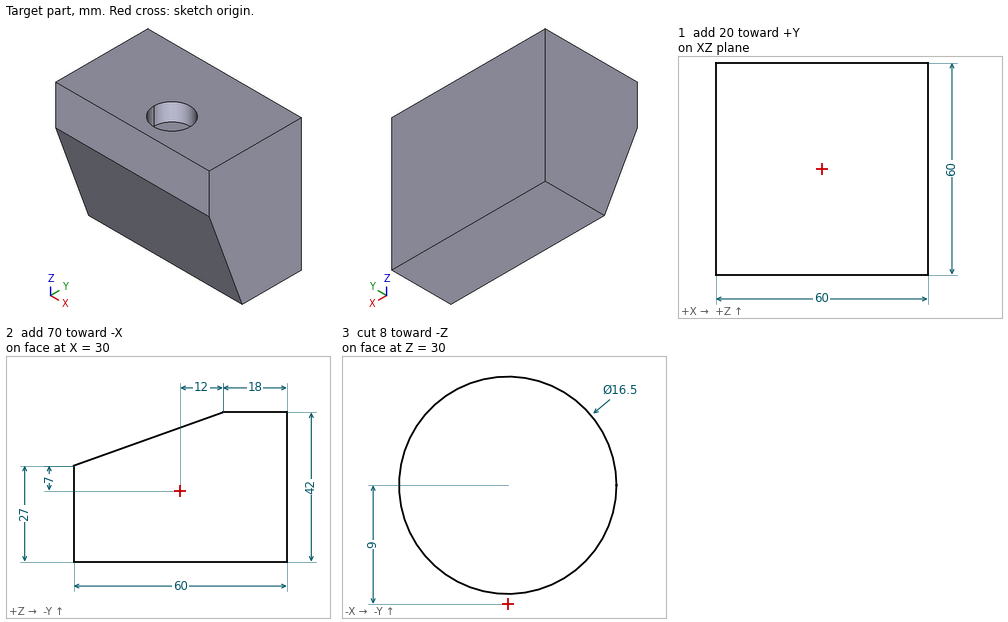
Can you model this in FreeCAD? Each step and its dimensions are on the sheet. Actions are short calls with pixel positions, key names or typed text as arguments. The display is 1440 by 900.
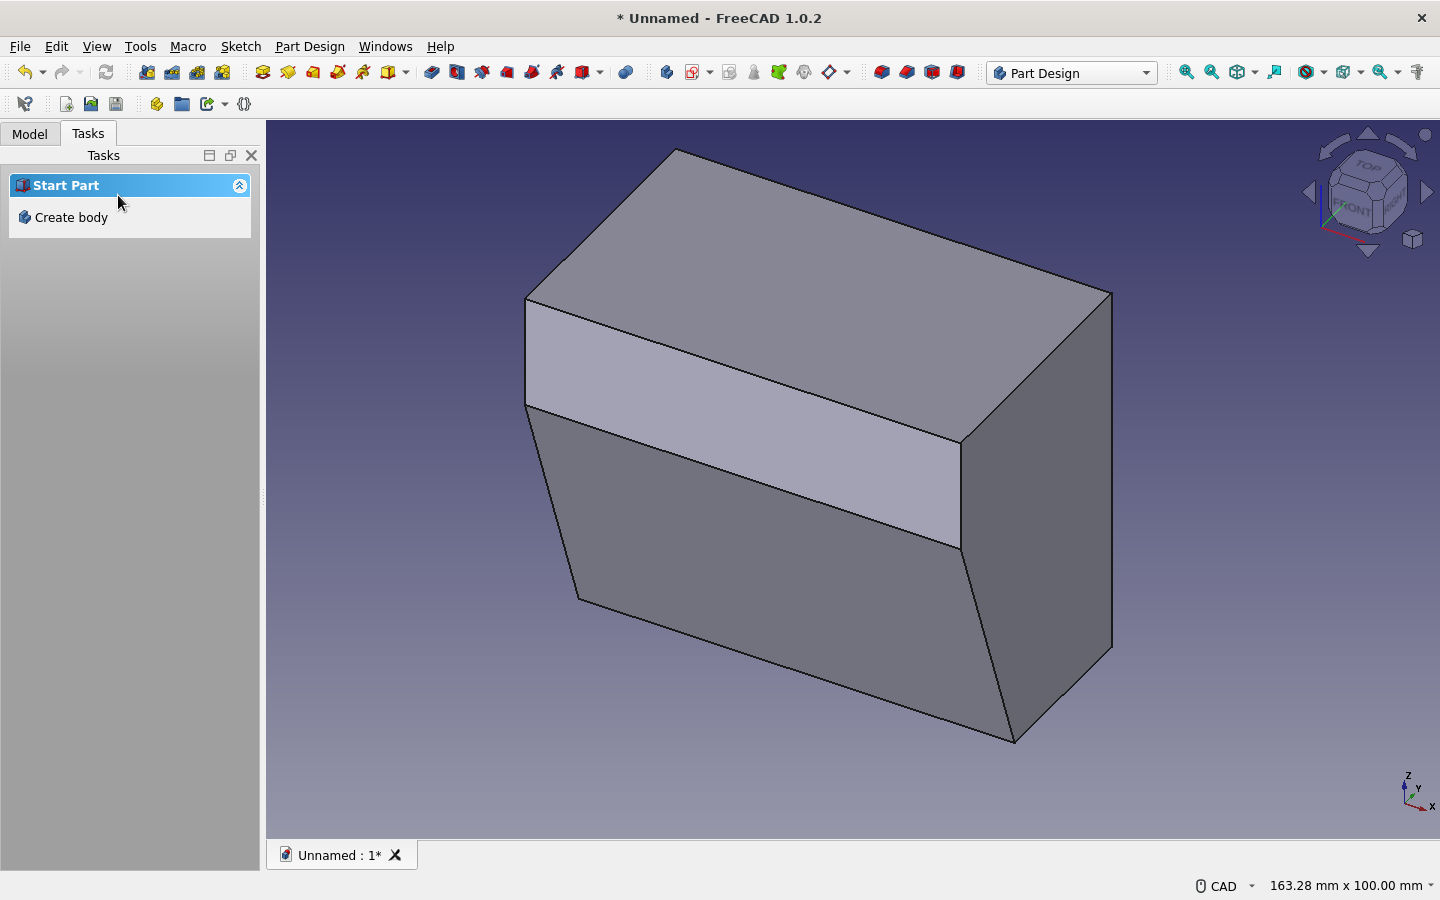
click(881, 316)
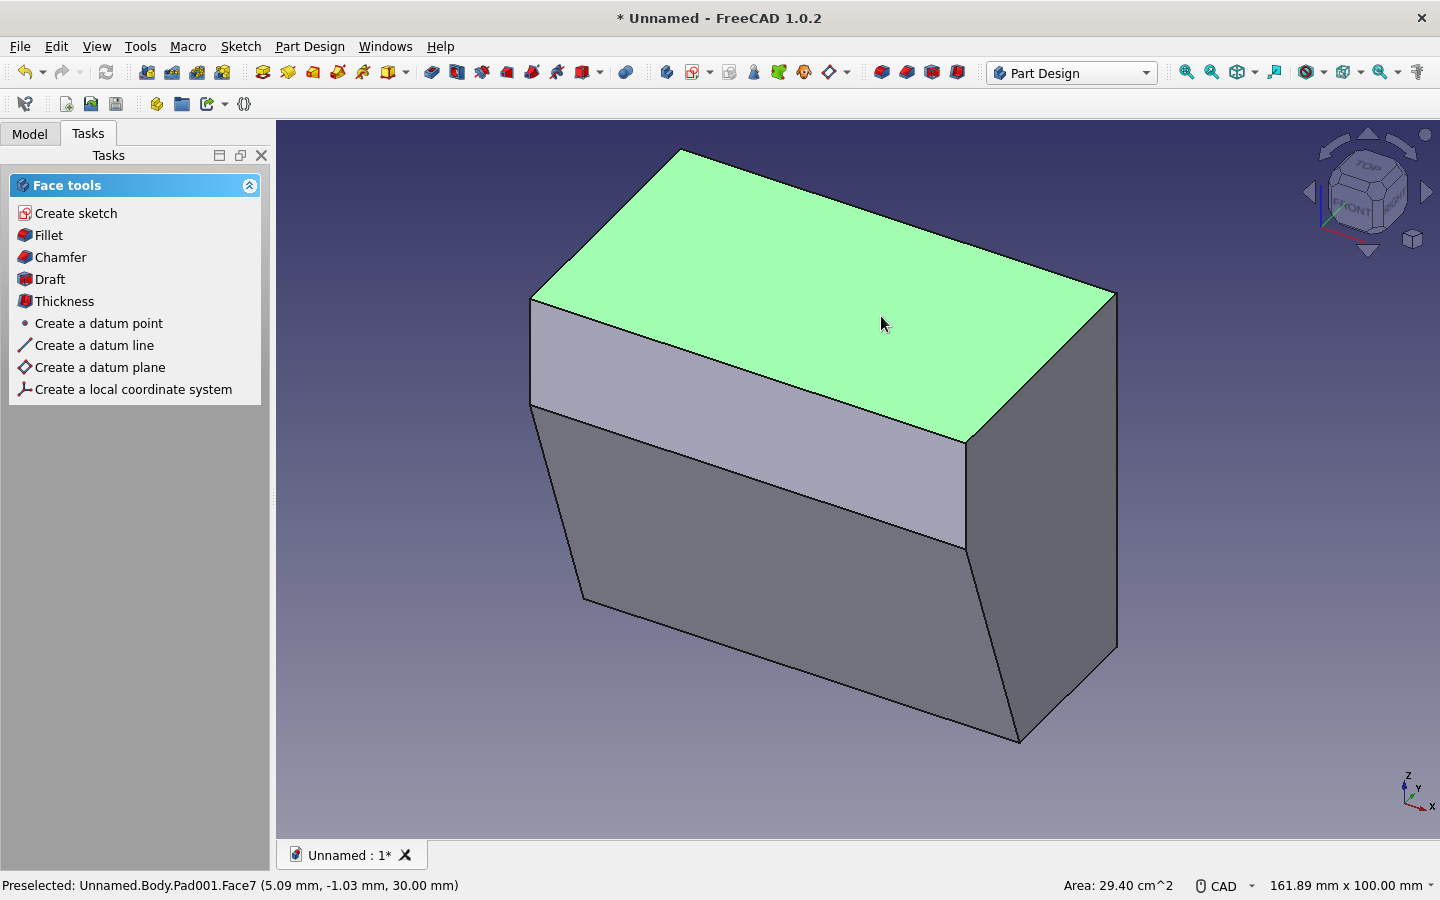
click(692, 72)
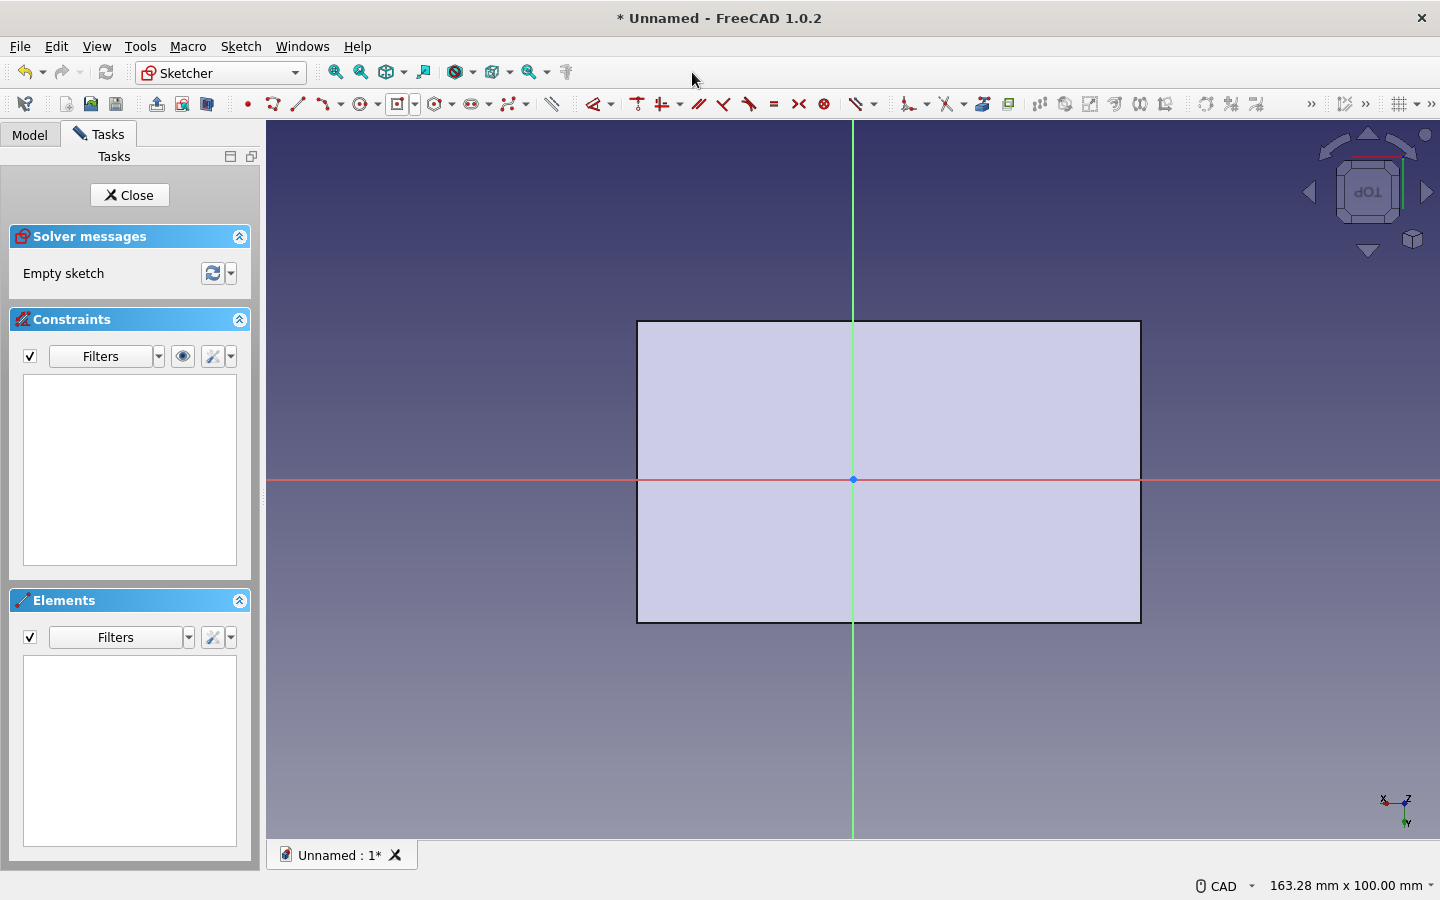
scroll(875, 397, up, 7)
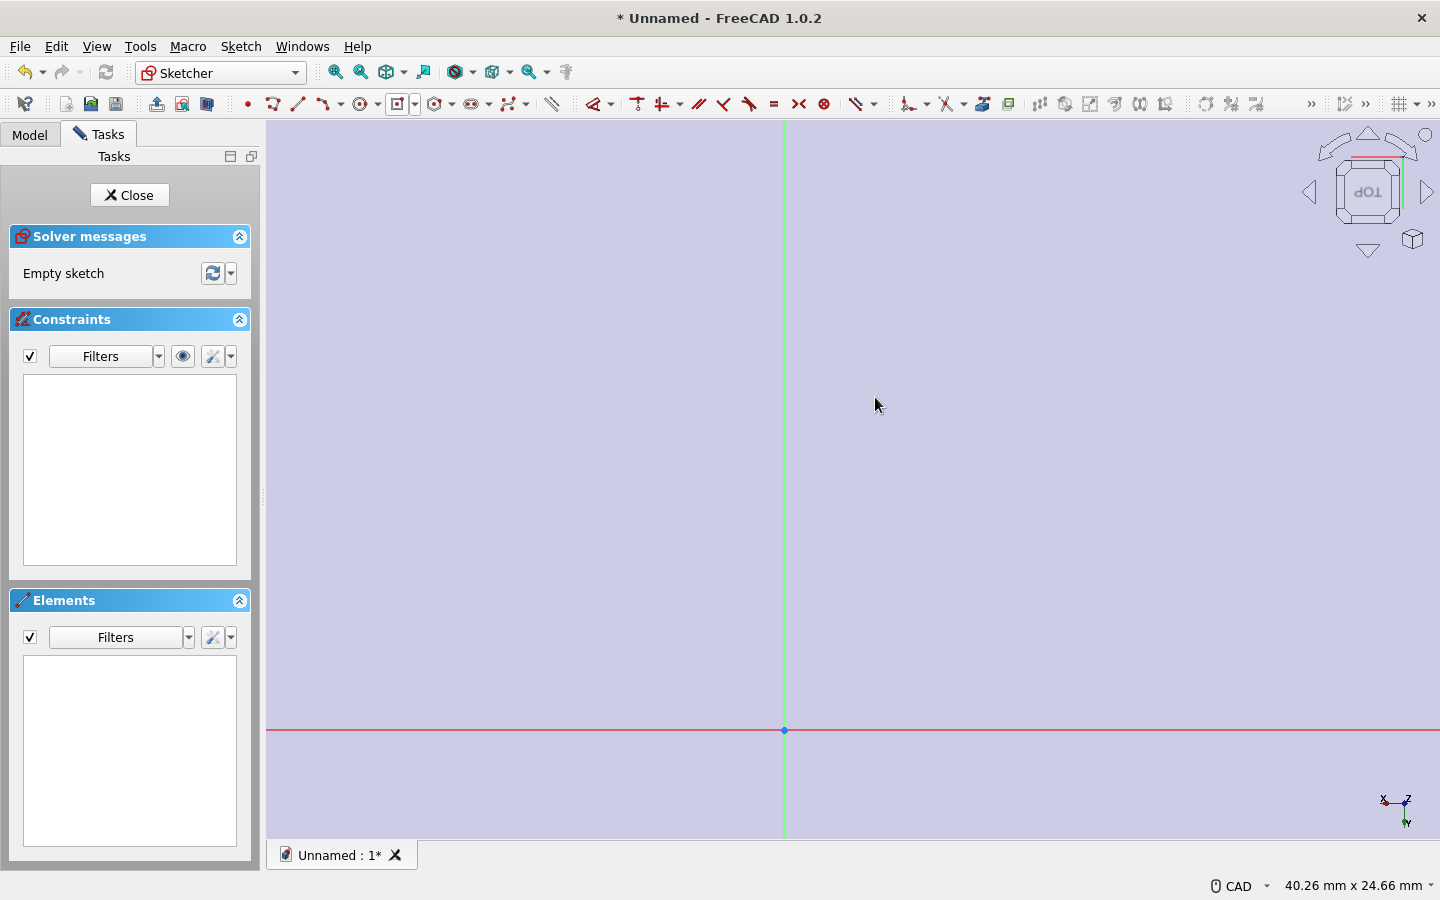
click(360, 104)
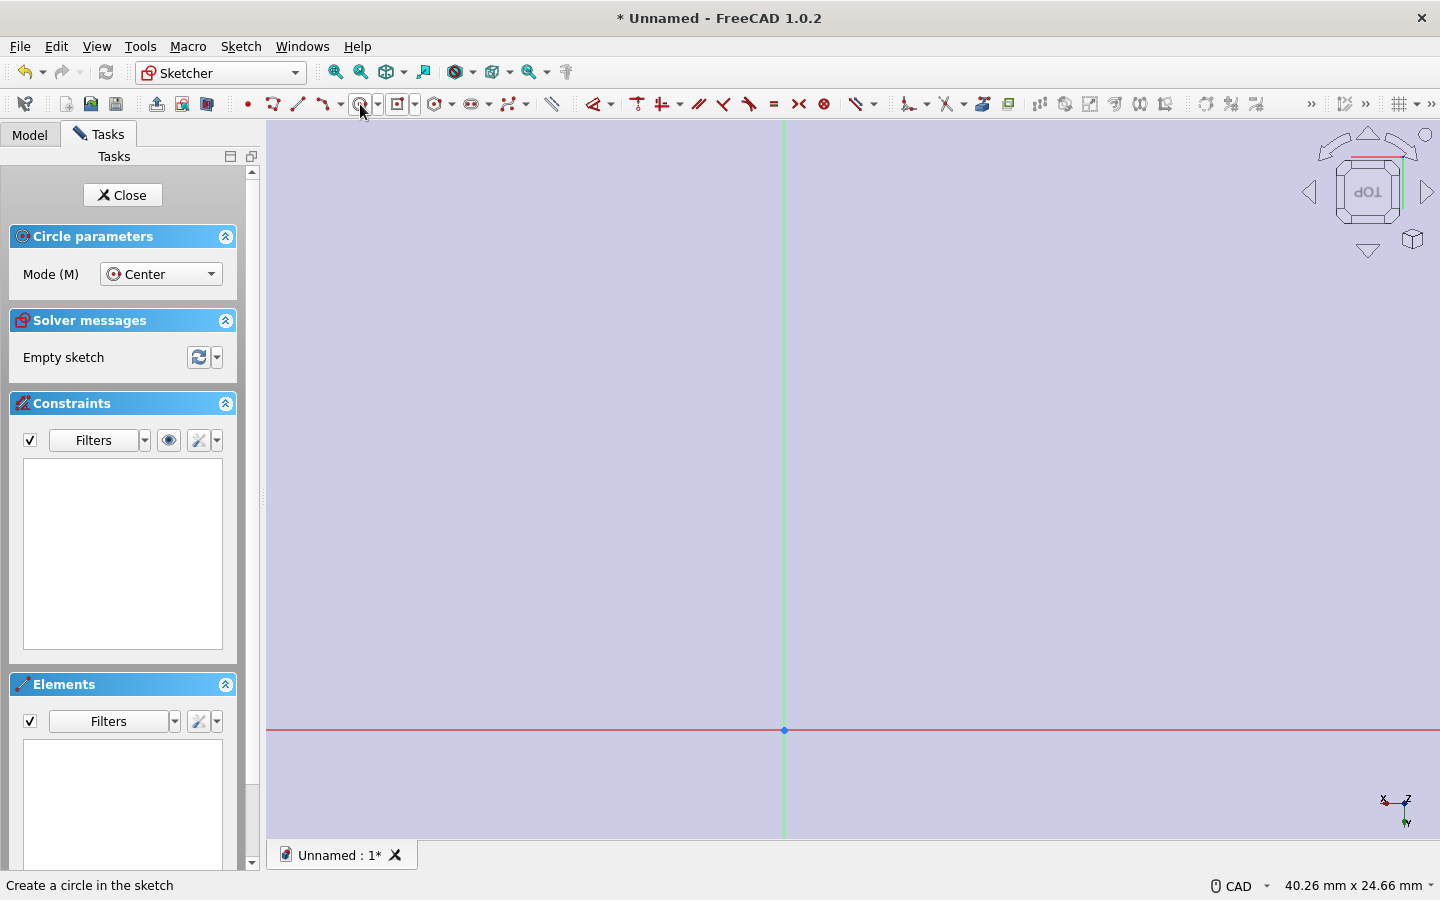
click(784, 468)
click(954, 298)
key(Escape)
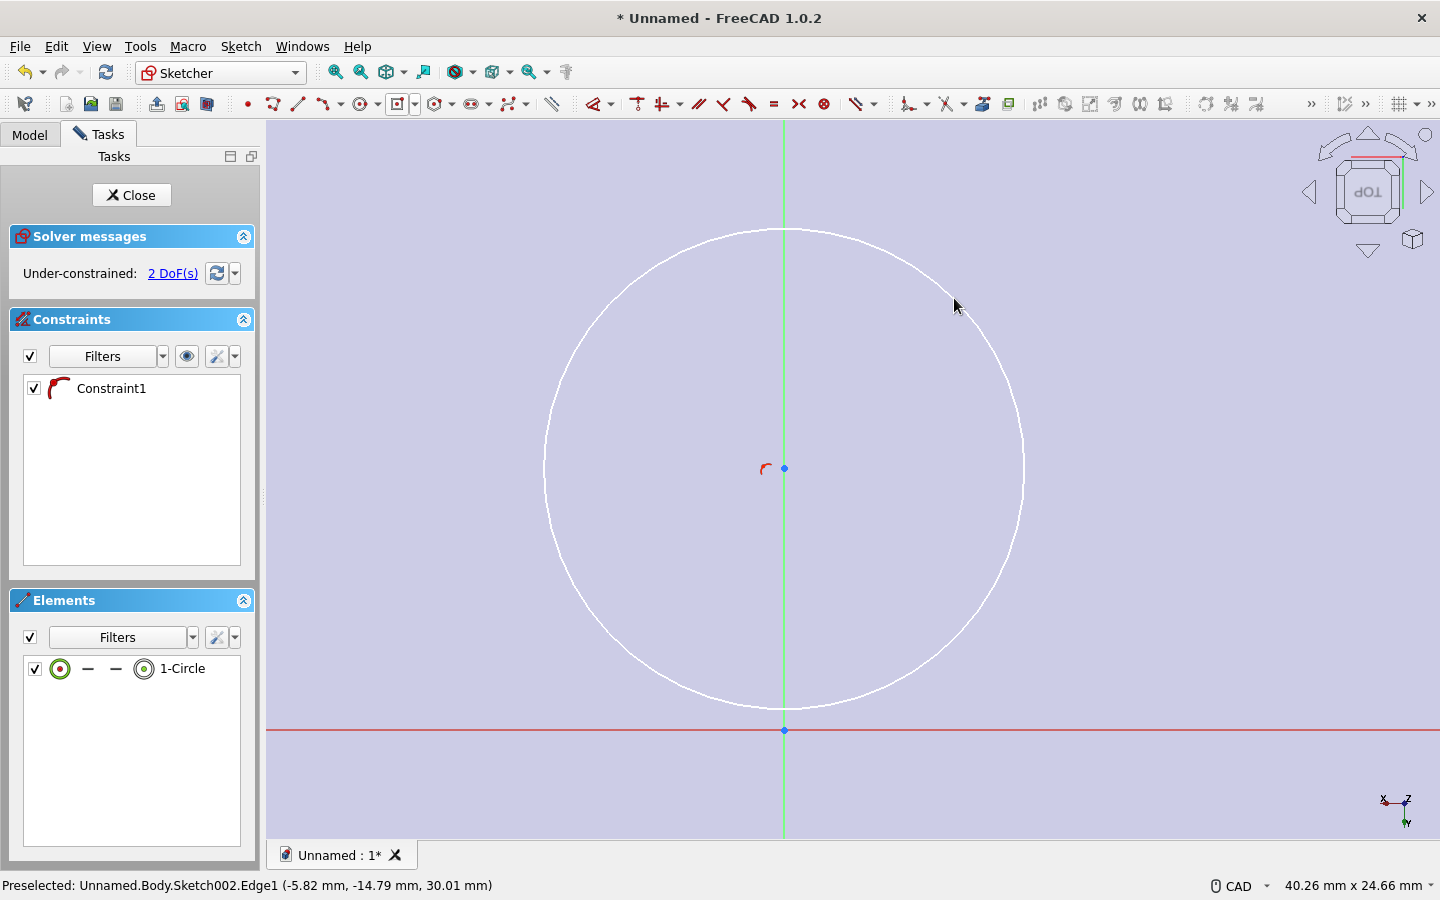
click(592, 104)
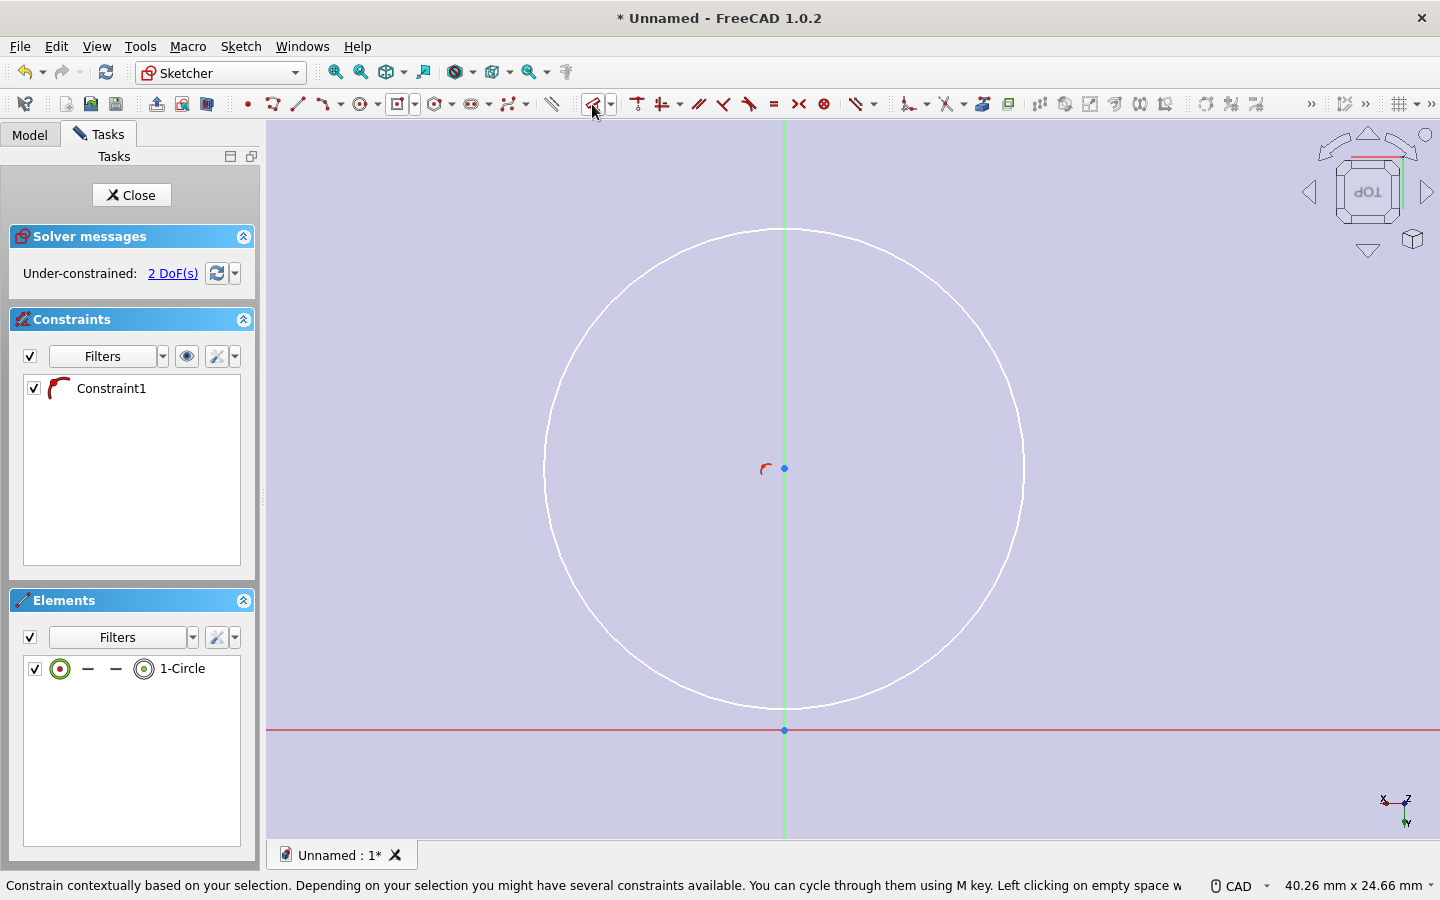
click(954, 299)
click(977, 276)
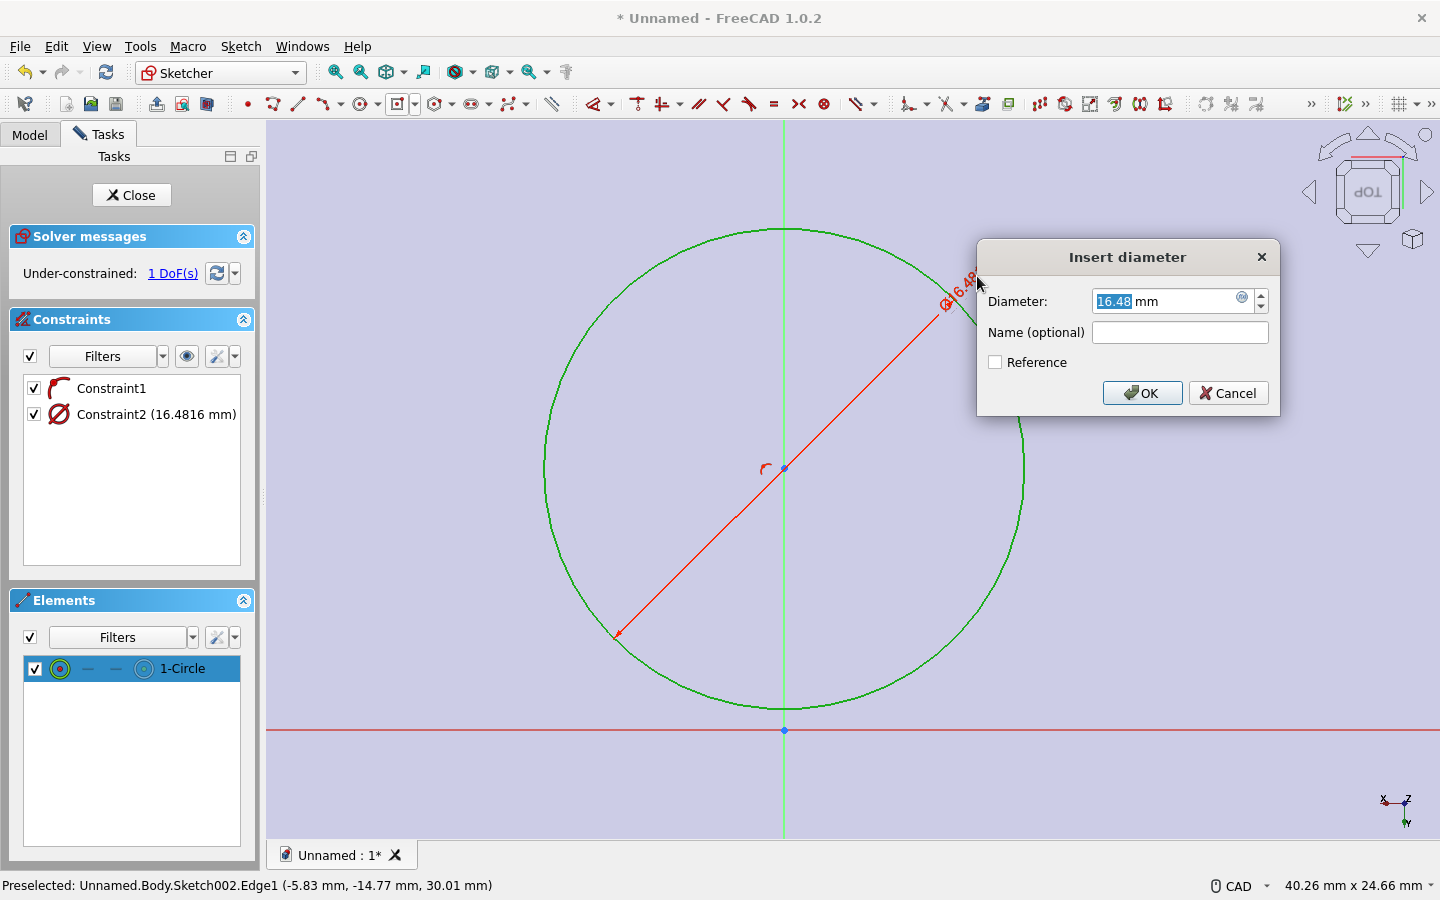
text(16.5)
key(Return)